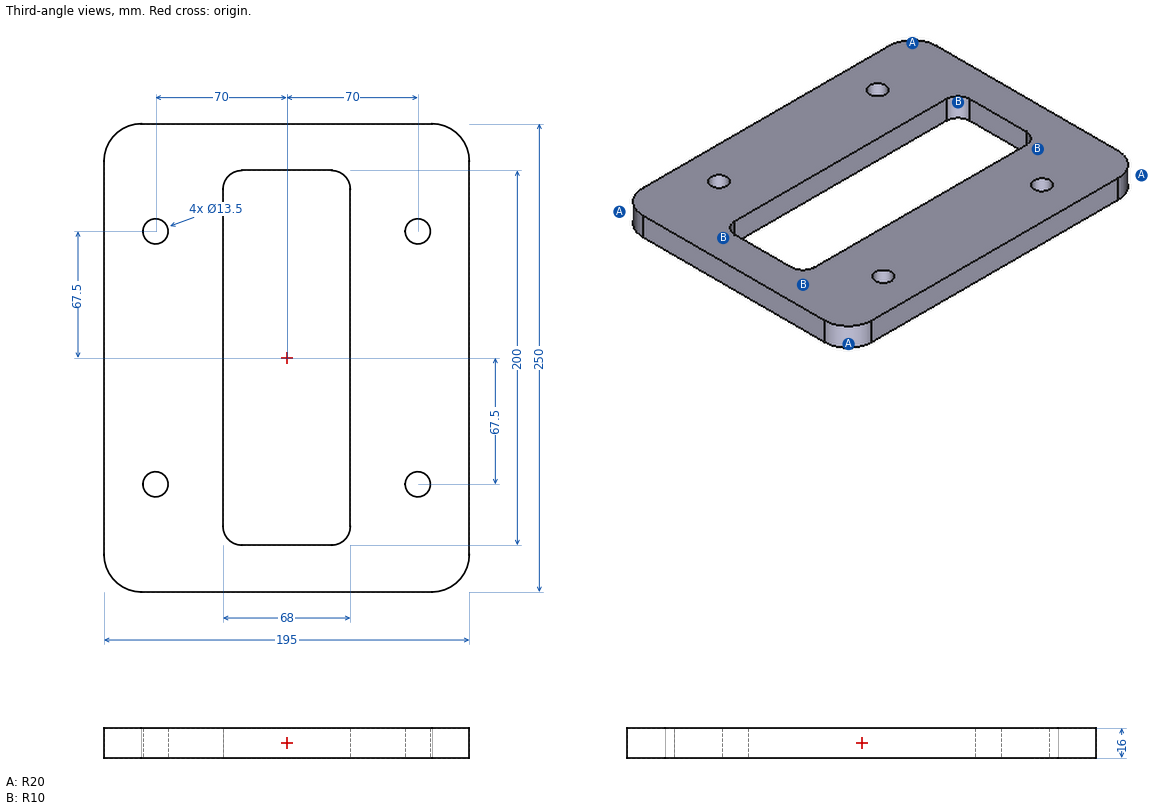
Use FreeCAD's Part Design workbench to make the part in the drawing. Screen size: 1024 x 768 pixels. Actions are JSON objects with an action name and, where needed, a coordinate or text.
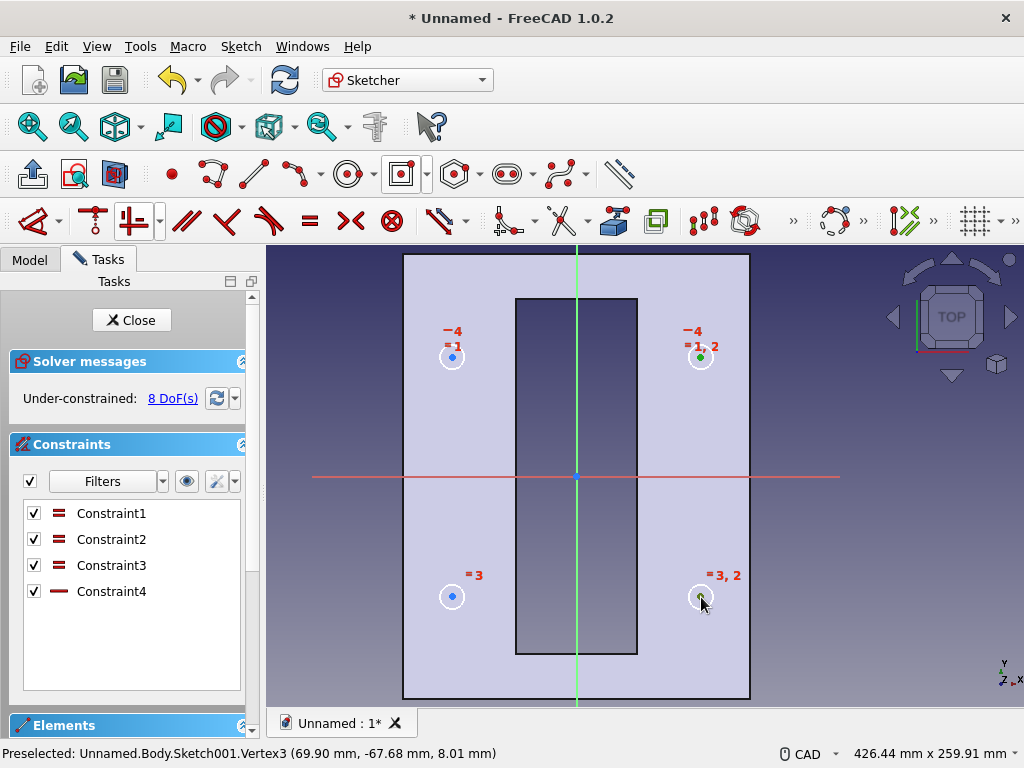
{"action": "key", "text": "v"}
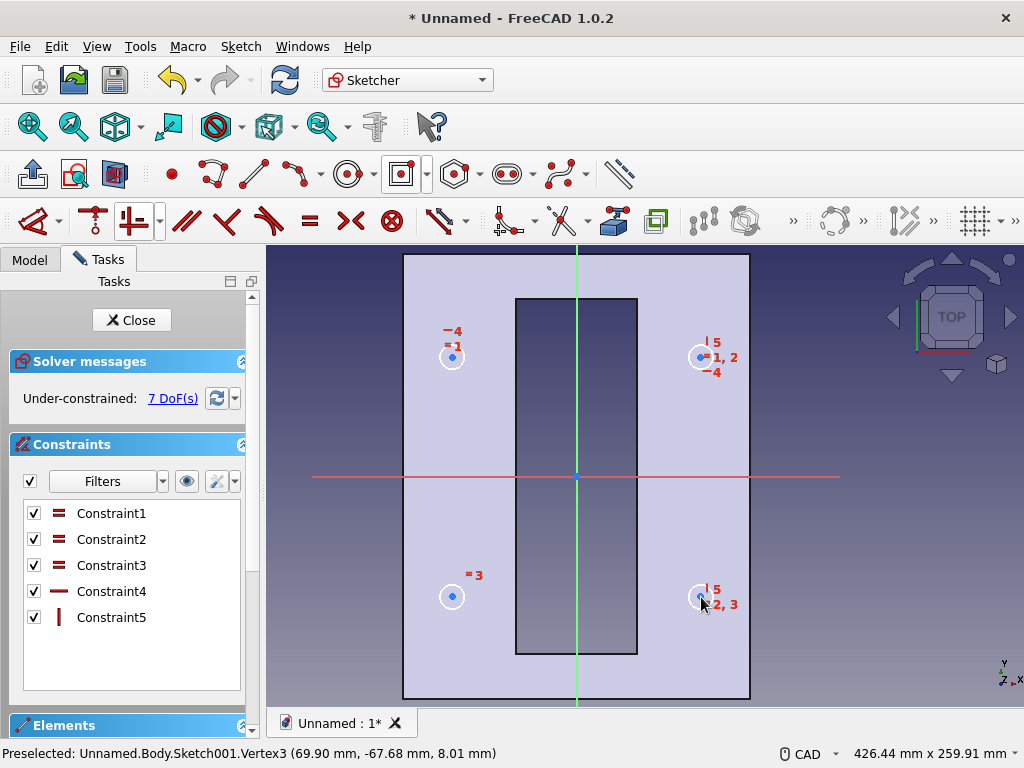
{"action": "left_click", "coordinate": [452, 357]}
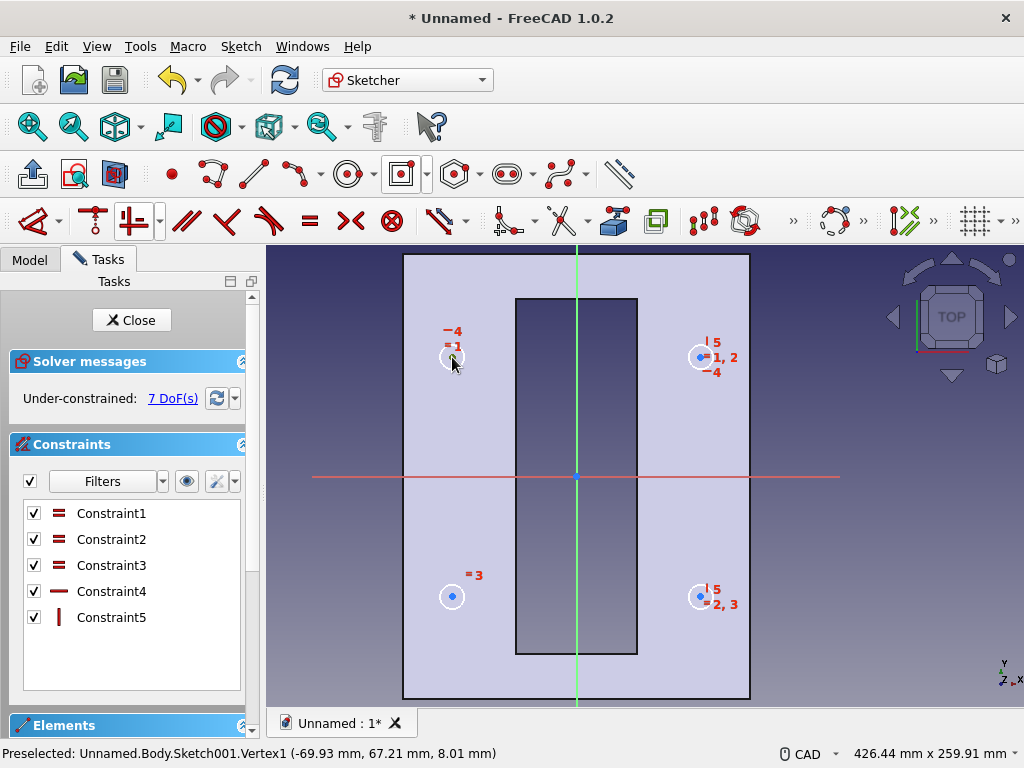
{"action": "left_click", "coordinate": [452, 597]}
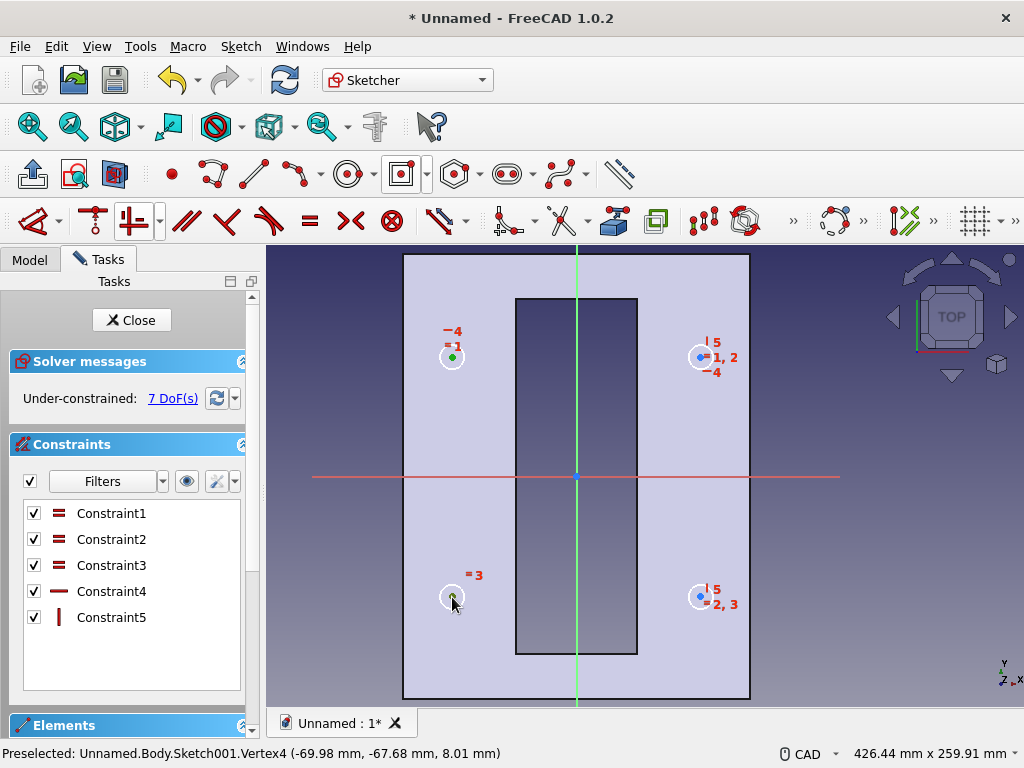
{"action": "left_click", "coordinate": [160, 222]}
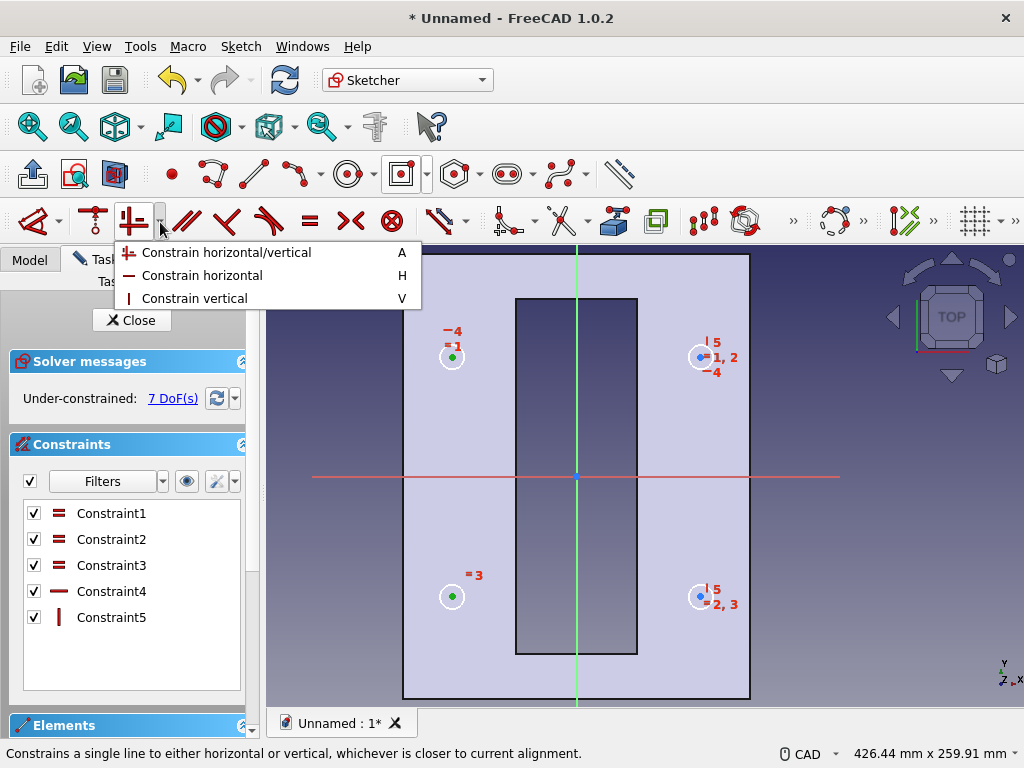
{"action": "left_click", "coordinate": [268, 298]}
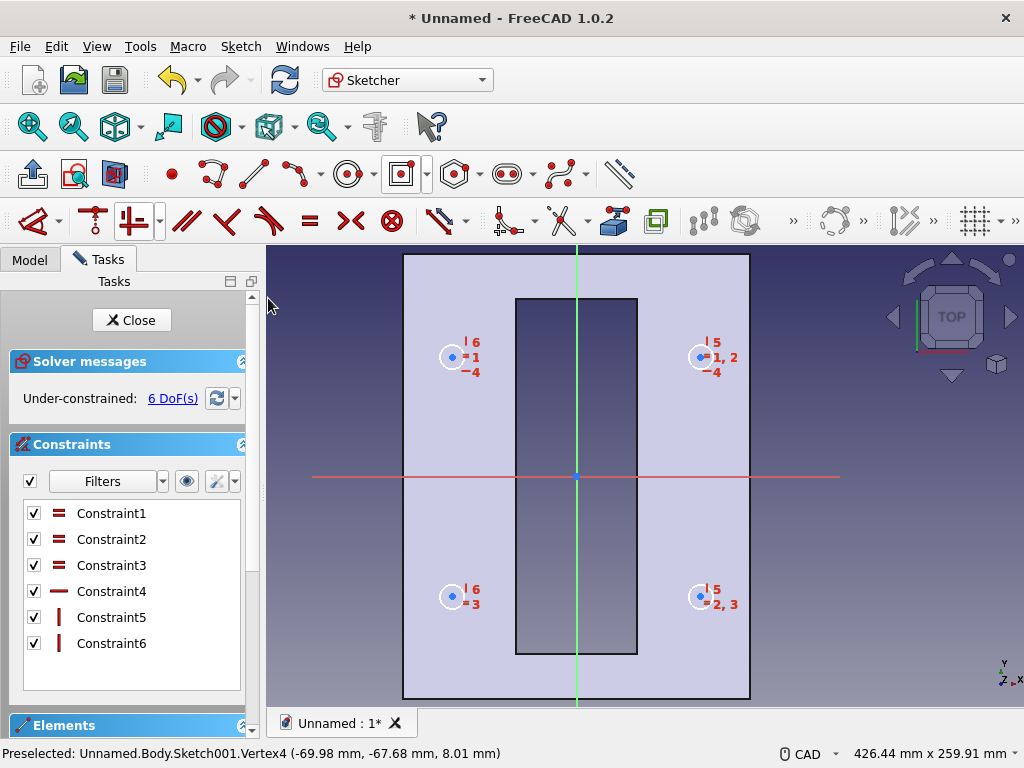
{"action": "left_click", "coordinate": [699, 599]}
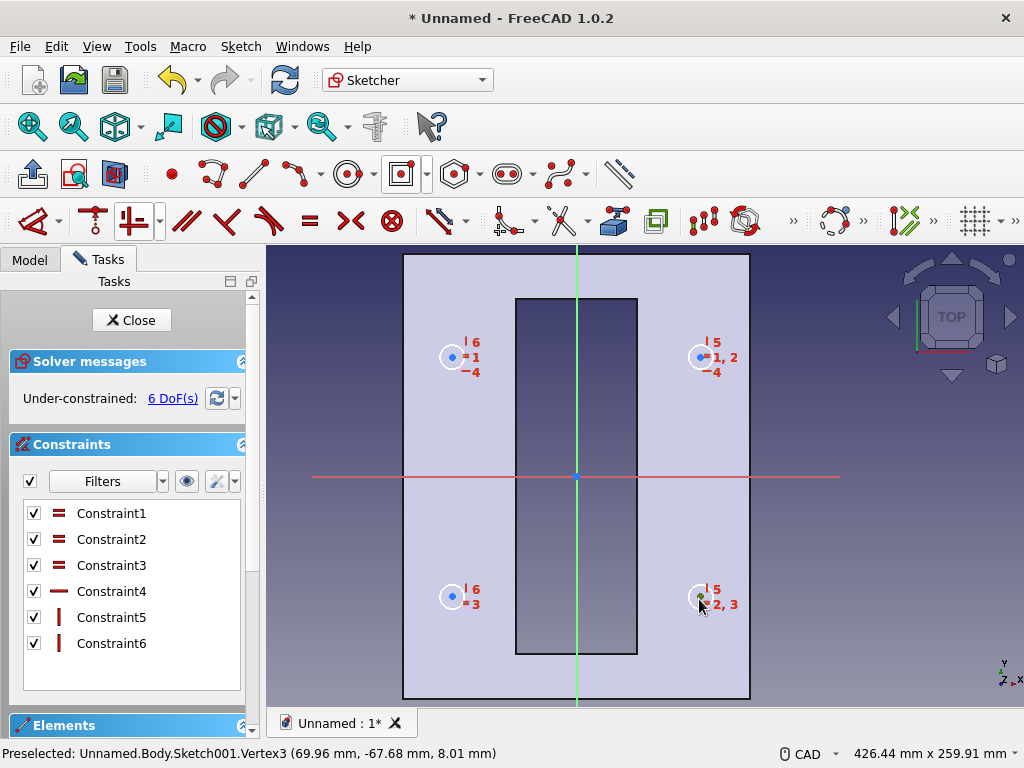
{"action": "left_click", "coordinate": [452, 597]}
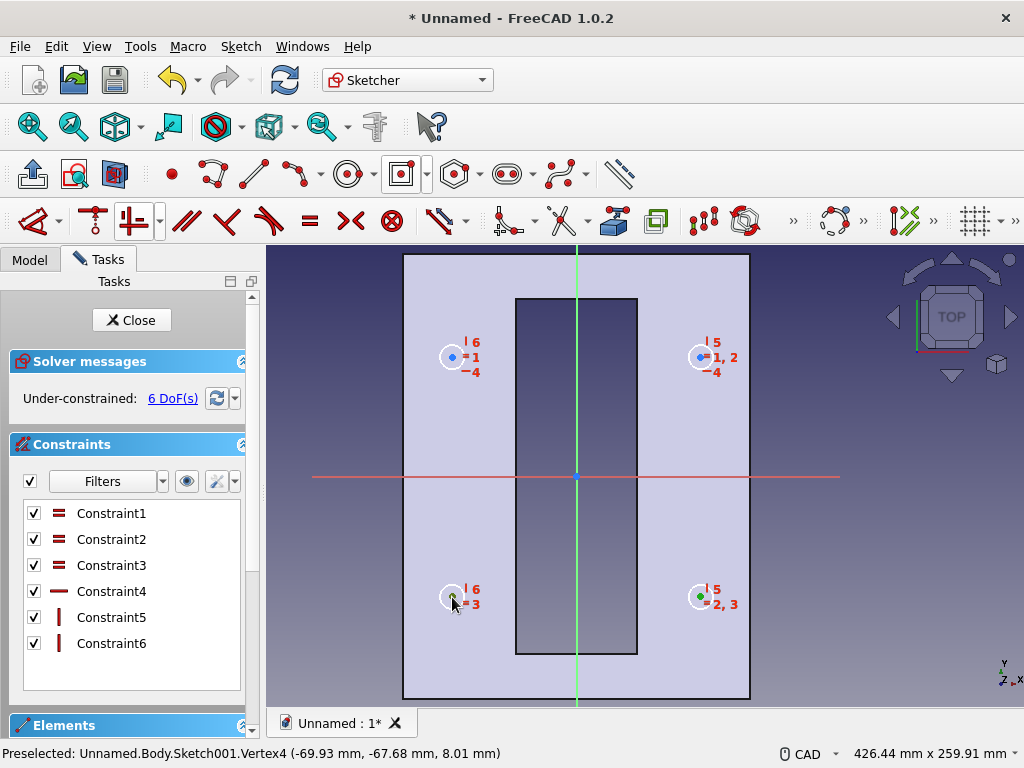
{"action": "key", "text": "h"}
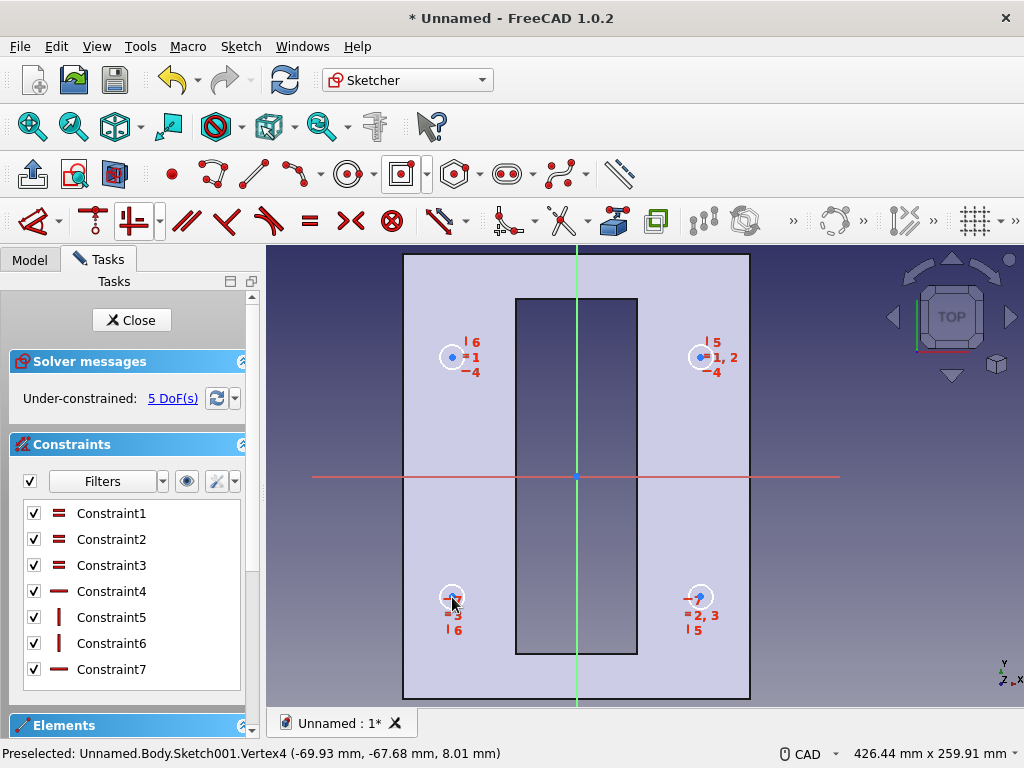
{"action": "left_click", "coordinate": [32, 222]}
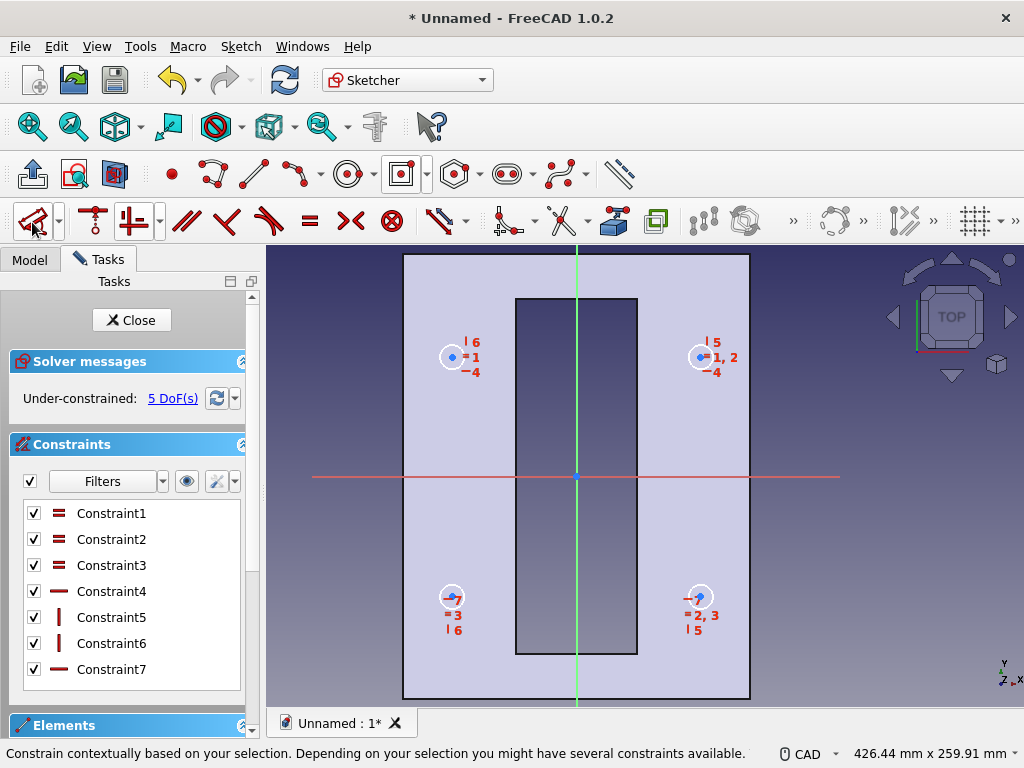
{"action": "scroll", "coordinate": [461, 349], "scroll_direction": "up", "scroll_amount": 3}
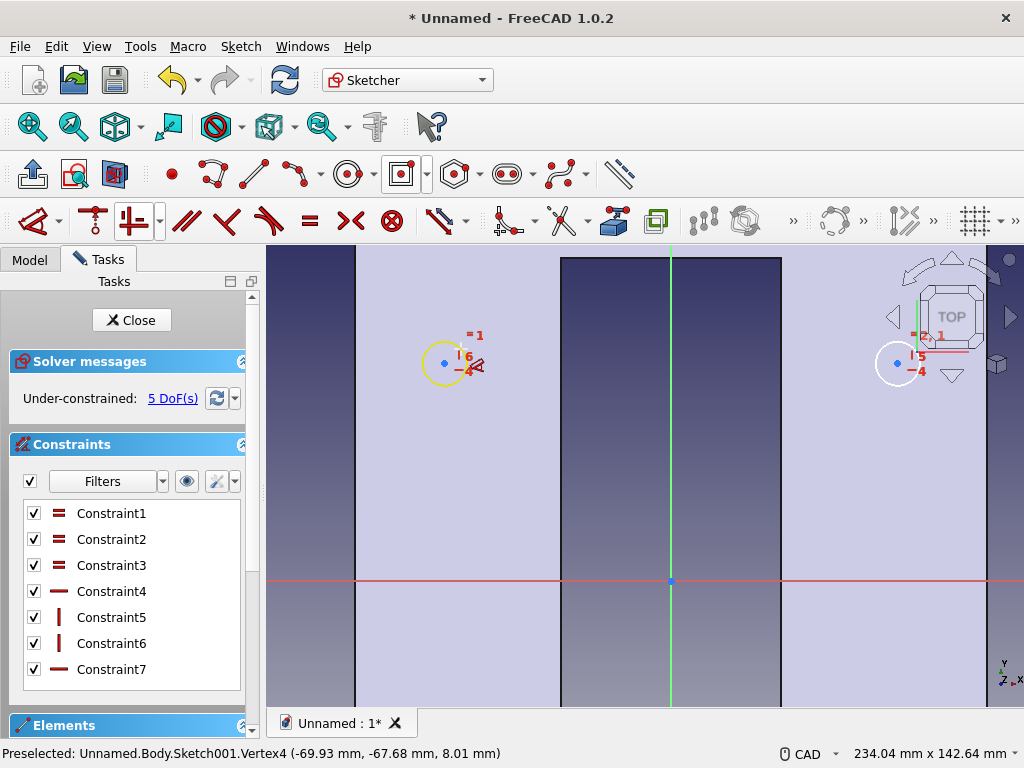
{"action": "left_click", "coordinate": [460, 348]}
{"action": "left_click", "coordinate": [482, 325]}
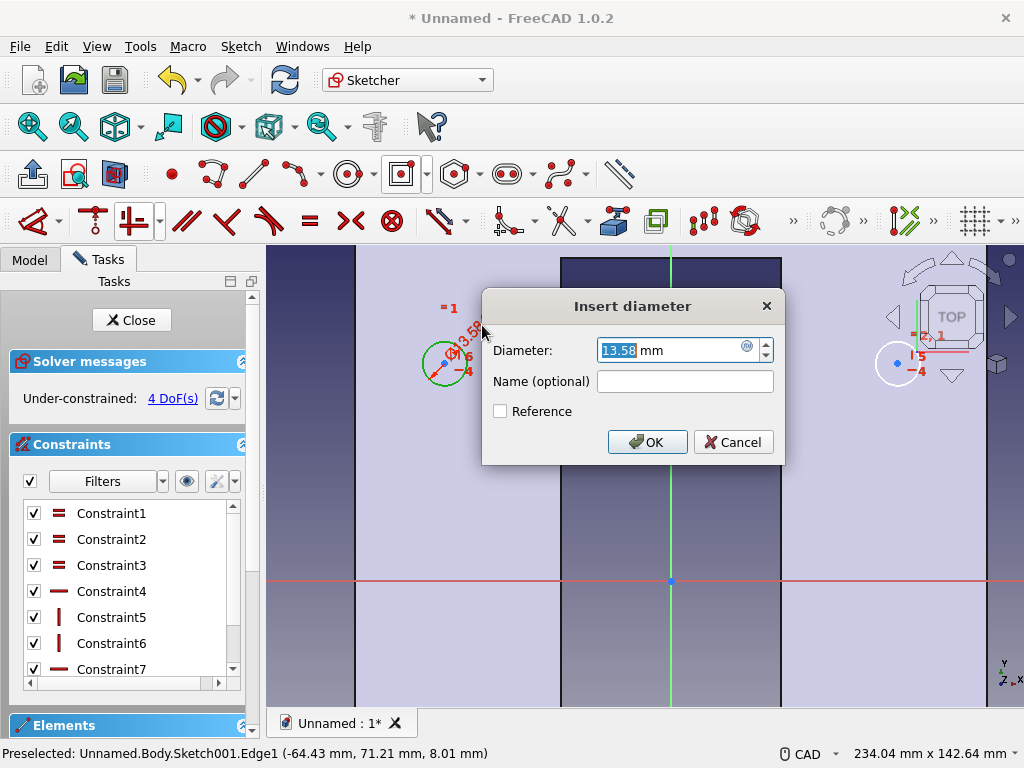
{"action": "type", "text": "13.5"}
{"action": "key", "text": "Return"}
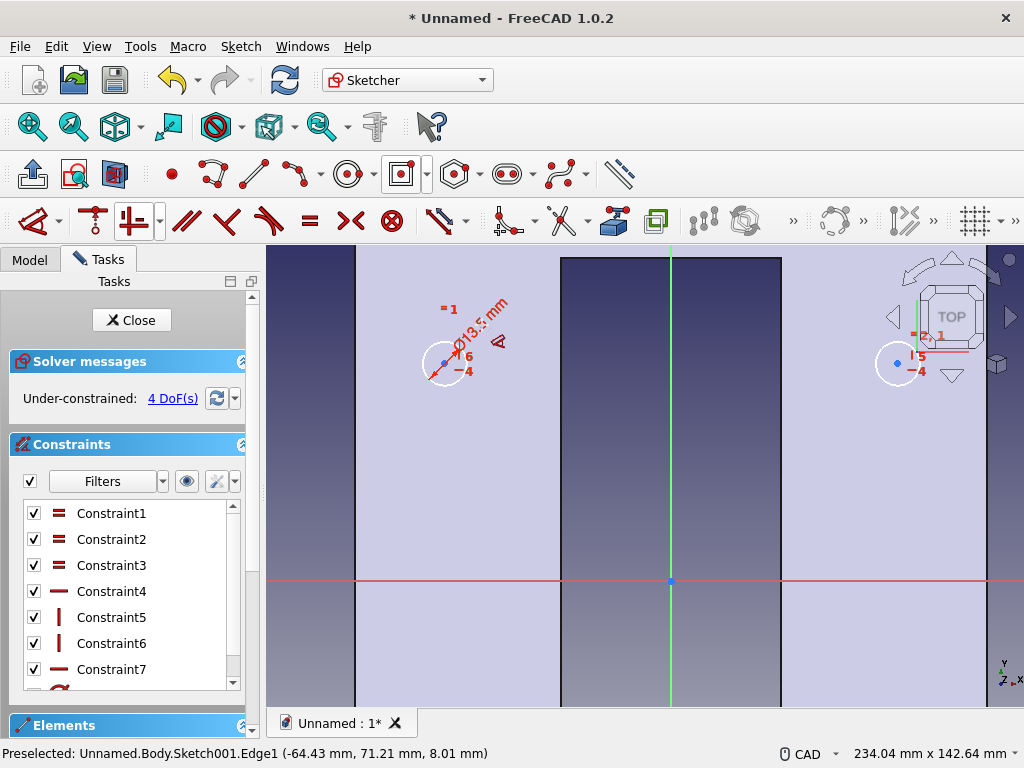
{"action": "left_click", "coordinate": [445, 364]}
{"action": "left_click", "coordinate": [558, 330]}